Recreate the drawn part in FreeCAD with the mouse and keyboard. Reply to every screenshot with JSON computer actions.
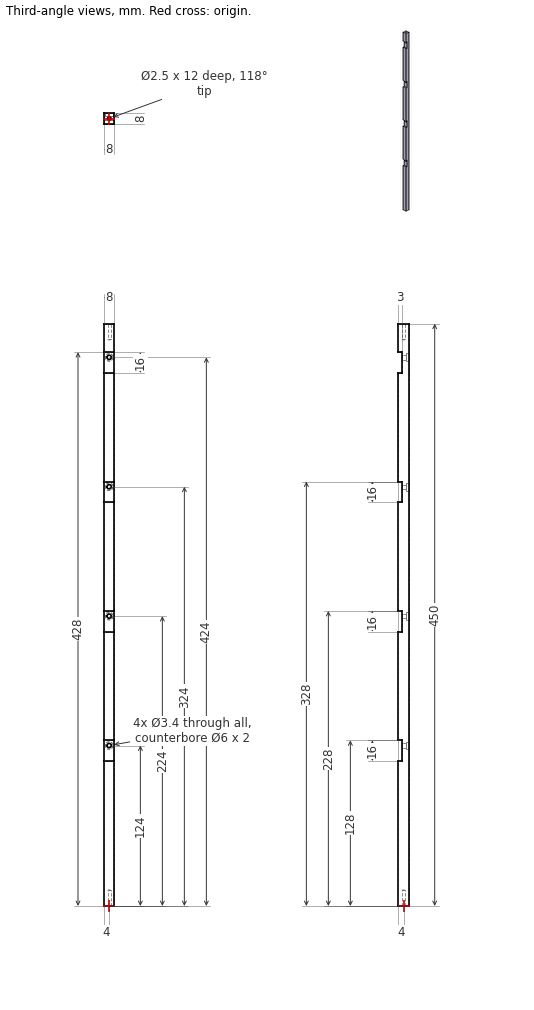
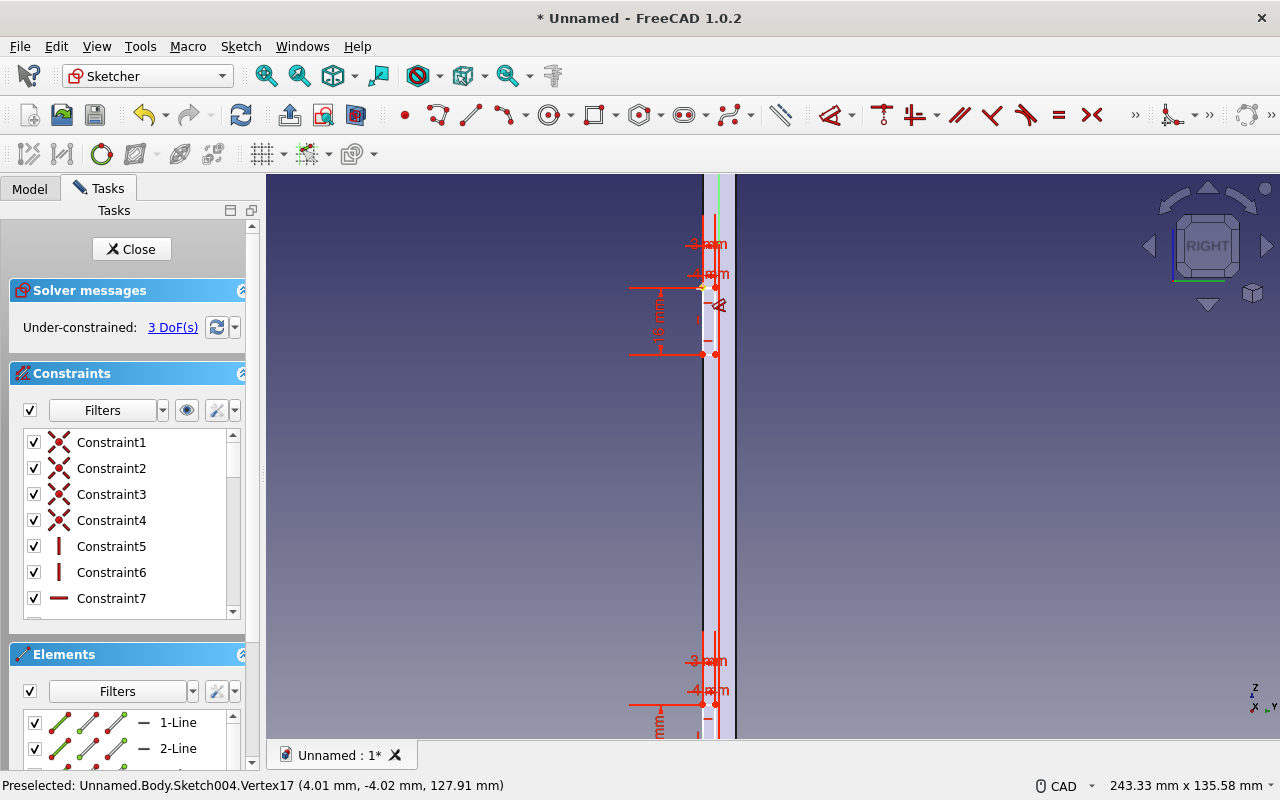
{"action": "left_click", "coordinate": [703, 288]}
{"action": "left_click", "coordinate": [753, 499]}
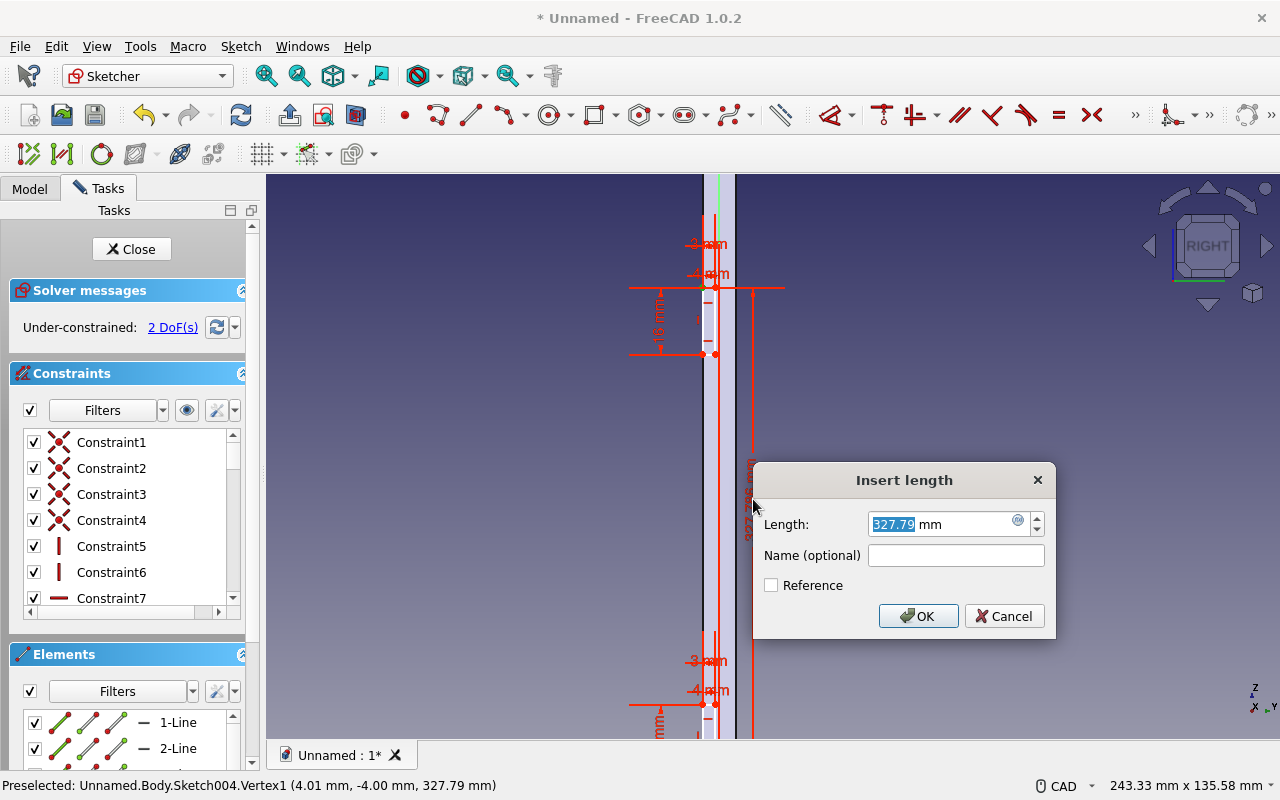
{"action": "type", "text": "328"}
{"action": "key", "text": "Return"}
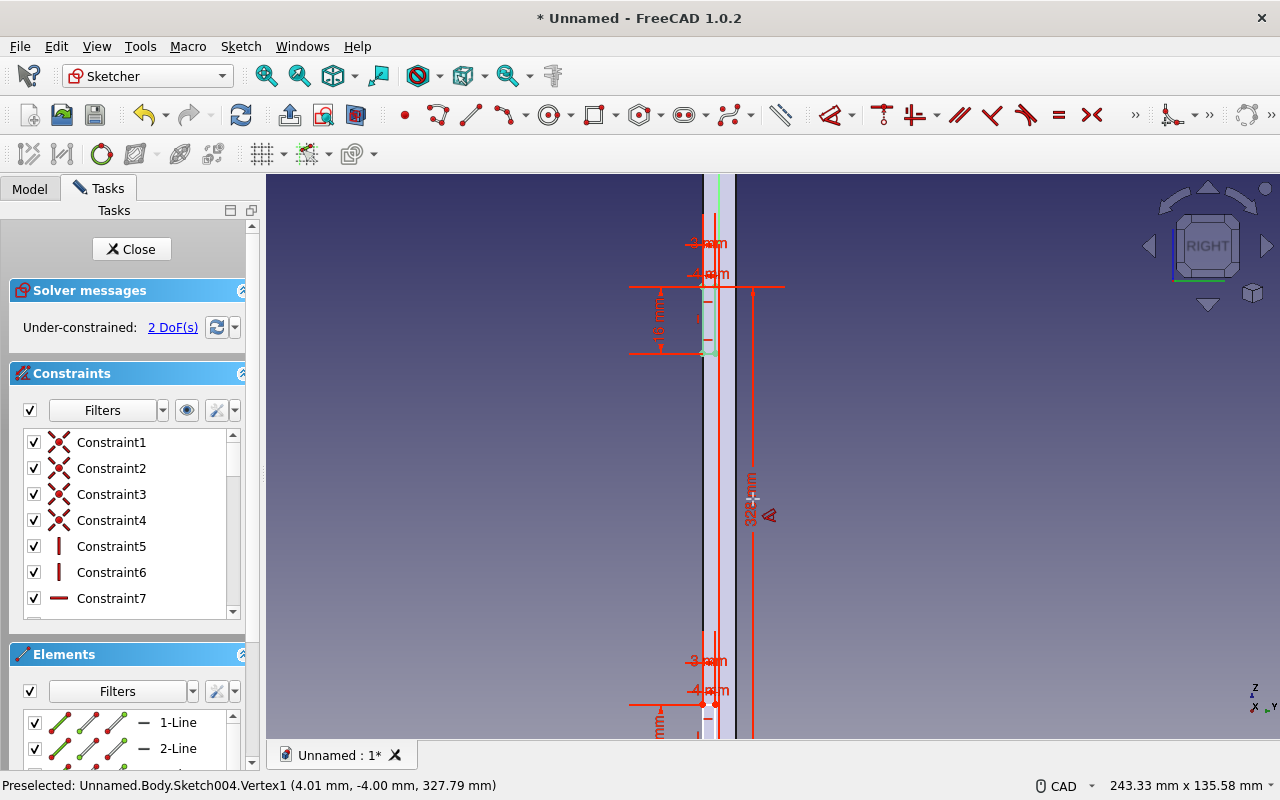
{"action": "left_click", "coordinate": [703, 705]}
{"action": "left_click", "coordinate": [801, 708]}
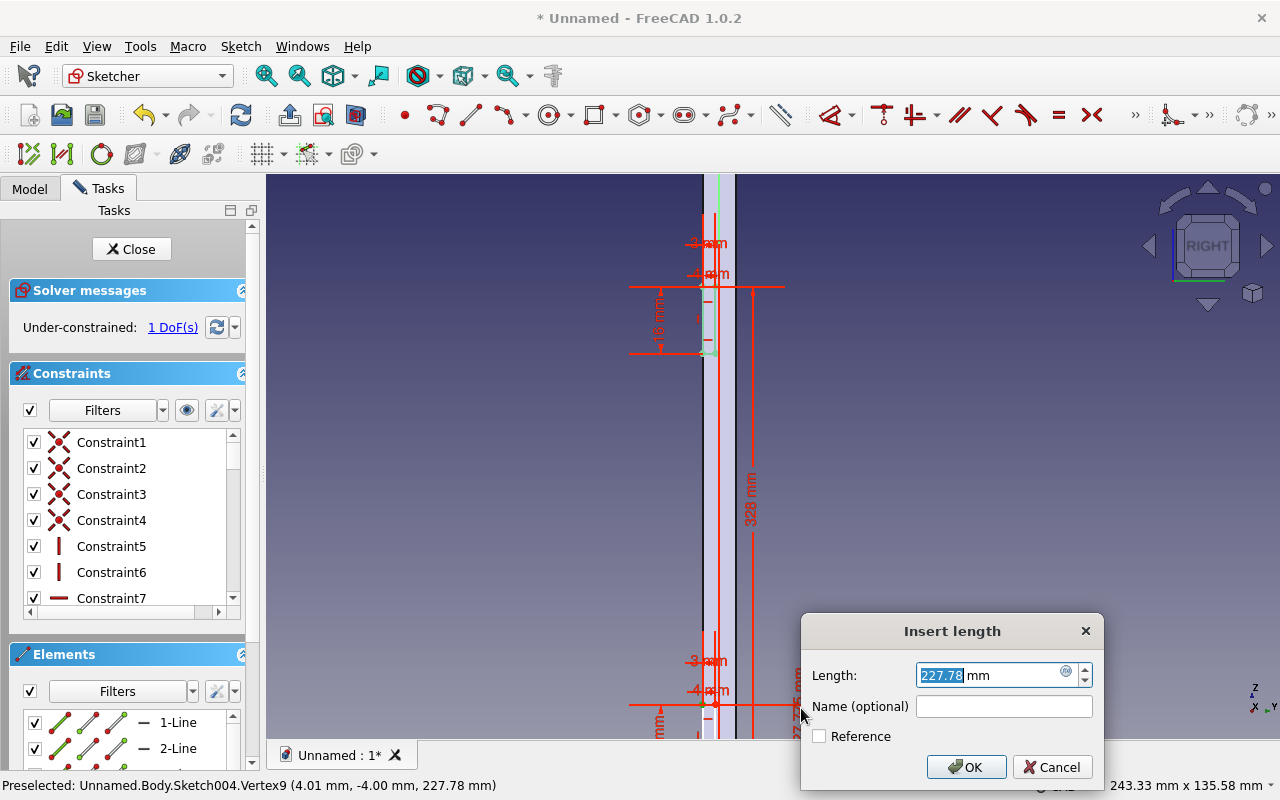
{"action": "type", "text": "228"}
{"action": "key", "text": "Return"}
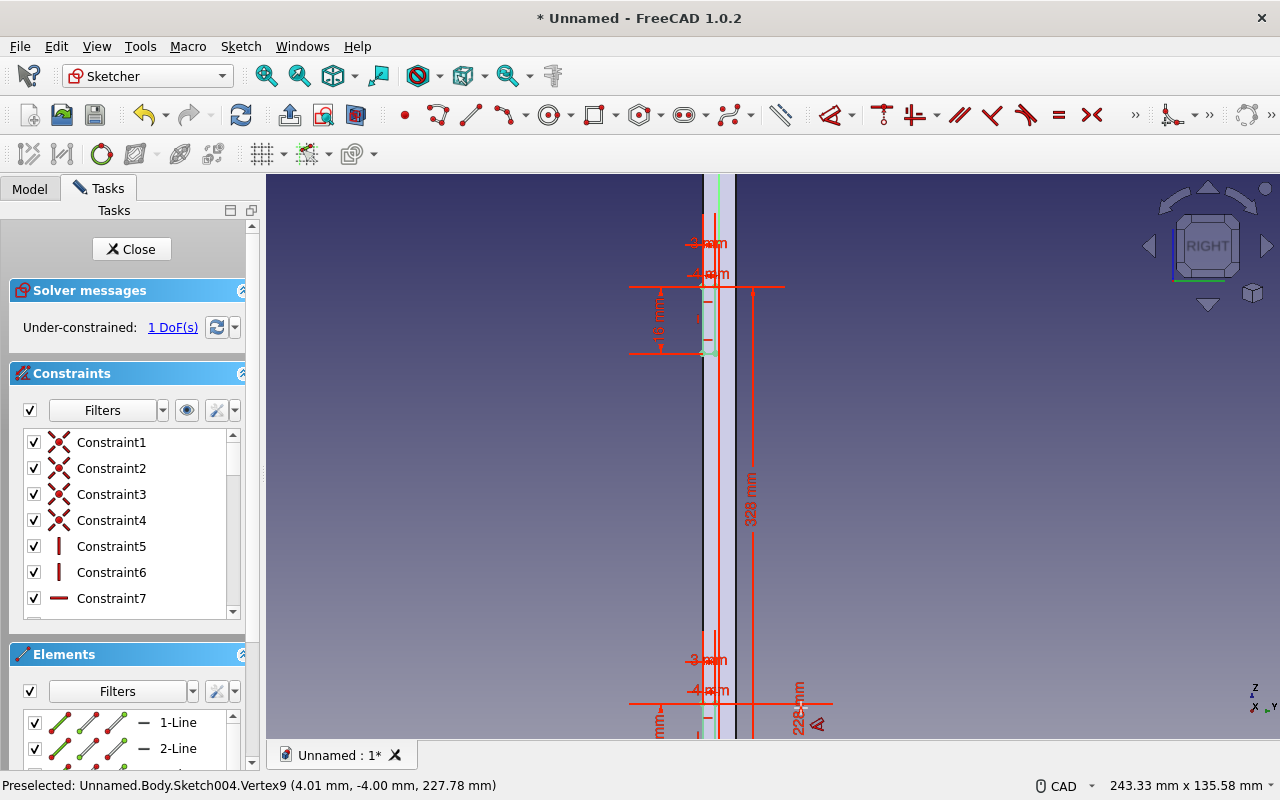
{"action": "scroll", "coordinate": [702, 288], "scroll_direction": "down", "scroll_amount": 7}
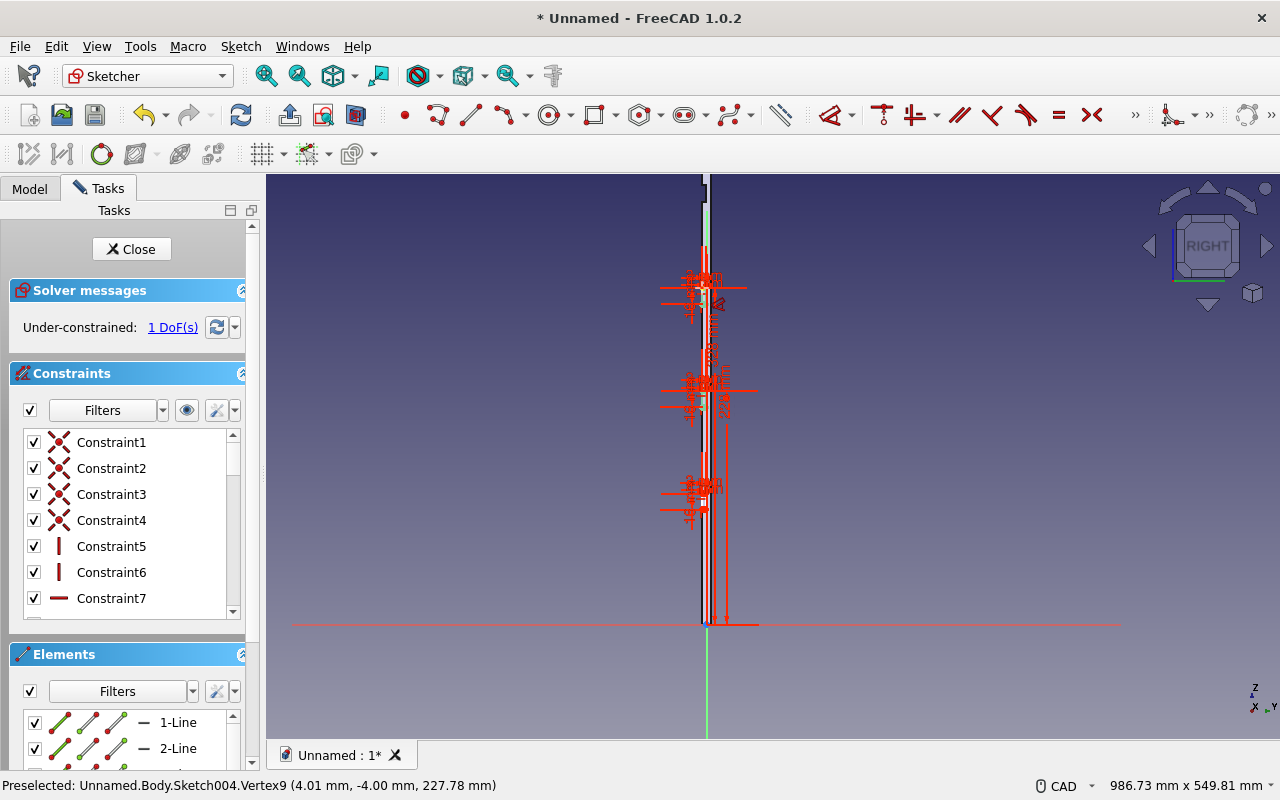
{"action": "scroll", "coordinate": [702, 494], "scroll_direction": "up", "scroll_amount": 7}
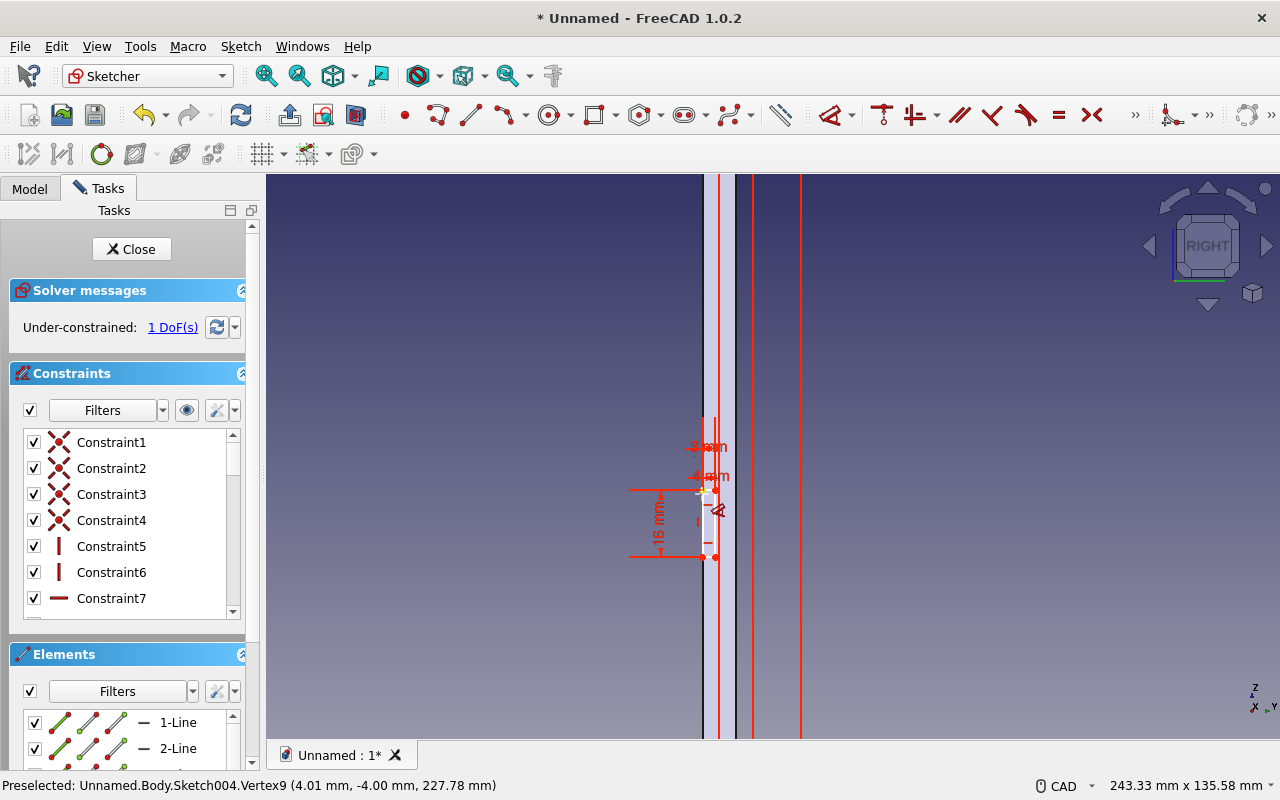
{"action": "left_click", "coordinate": [703, 490]}
{"action": "left_click", "coordinate": [753, 601]}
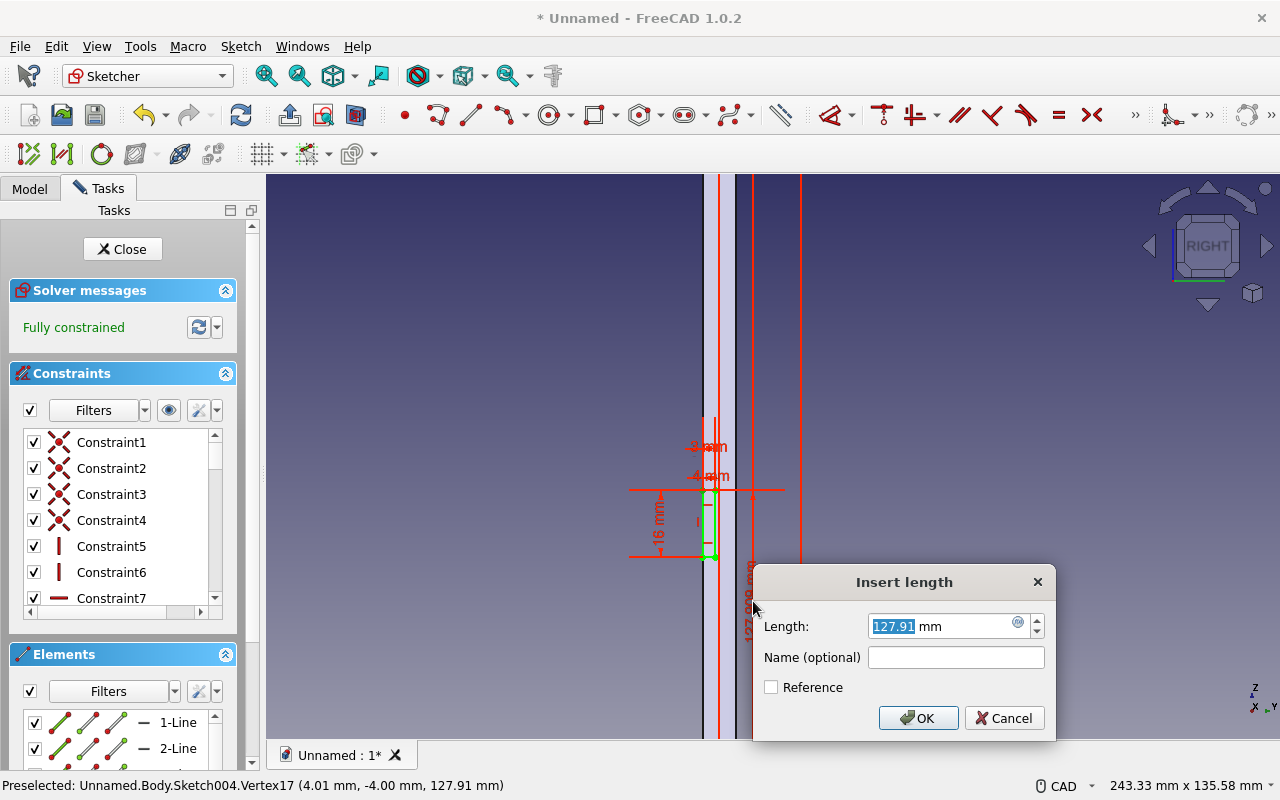
{"action": "type", "text": "128"}
{"action": "key", "text": "Return"}
{"action": "key", "text": "Escape"}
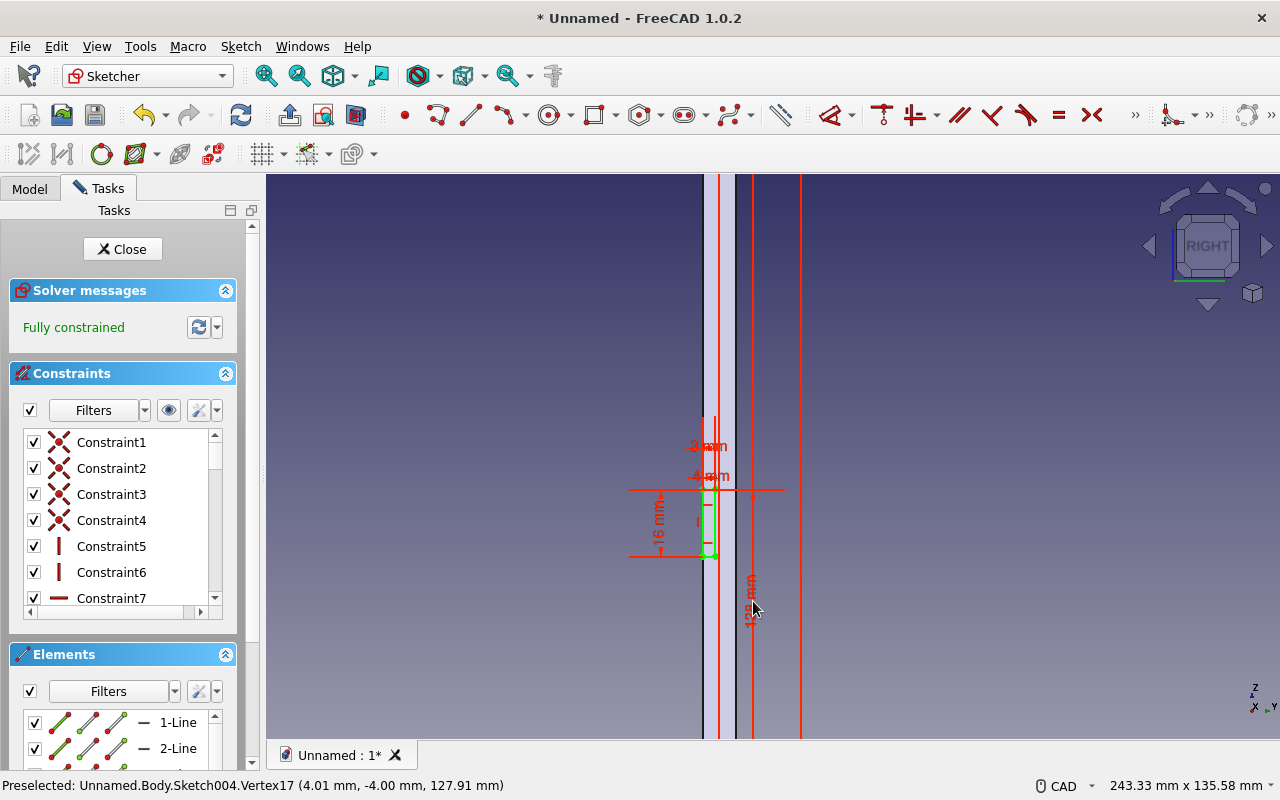
{"action": "left_click", "coordinate": [123, 249]}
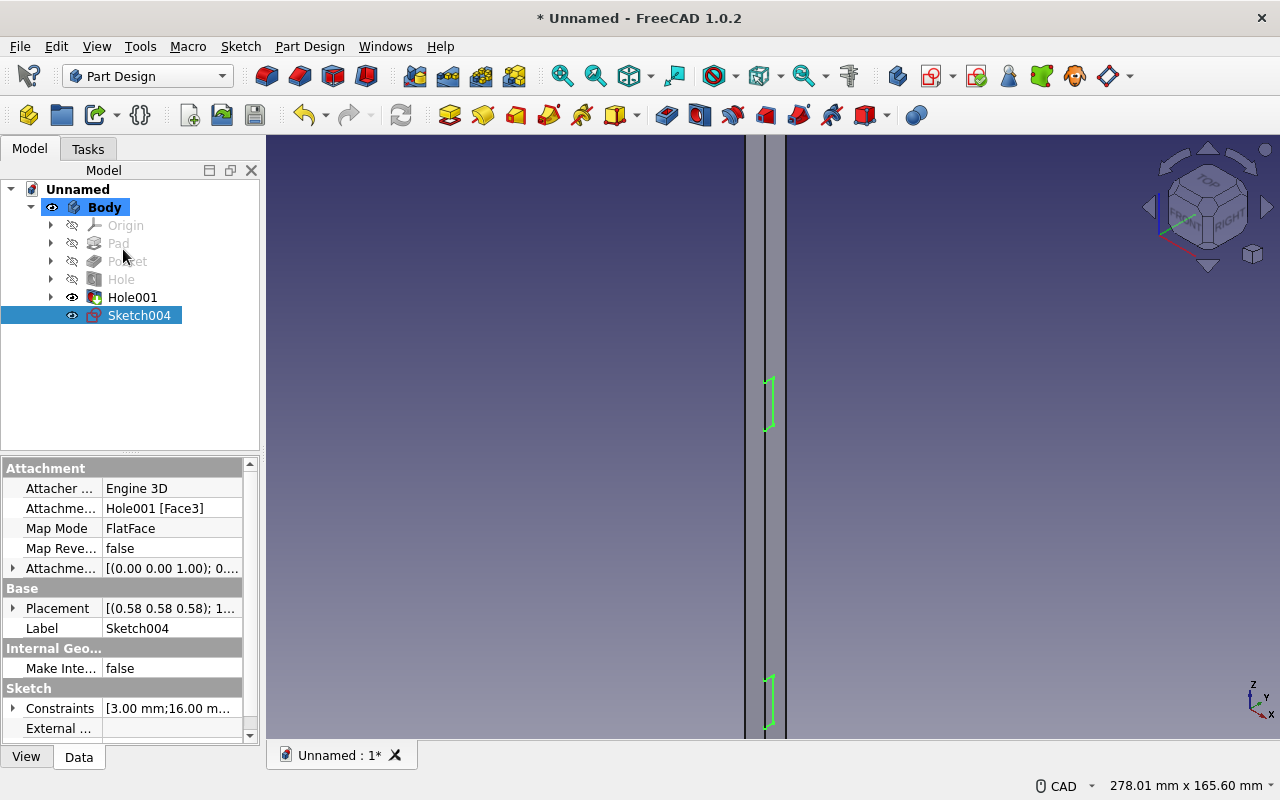
{"action": "left_click", "coordinate": [667, 116]}